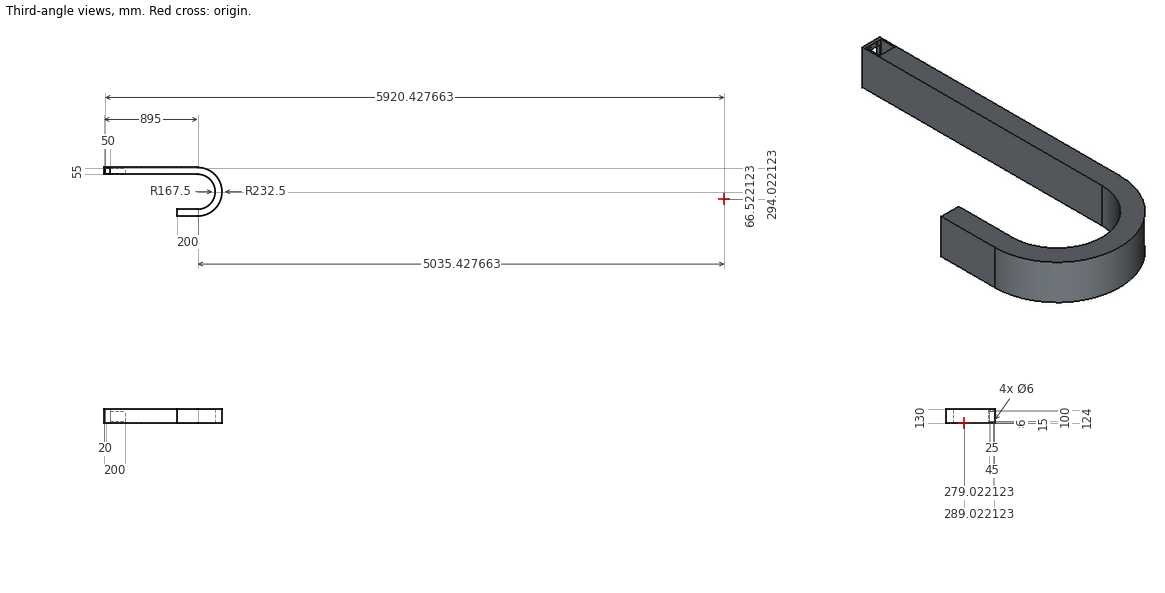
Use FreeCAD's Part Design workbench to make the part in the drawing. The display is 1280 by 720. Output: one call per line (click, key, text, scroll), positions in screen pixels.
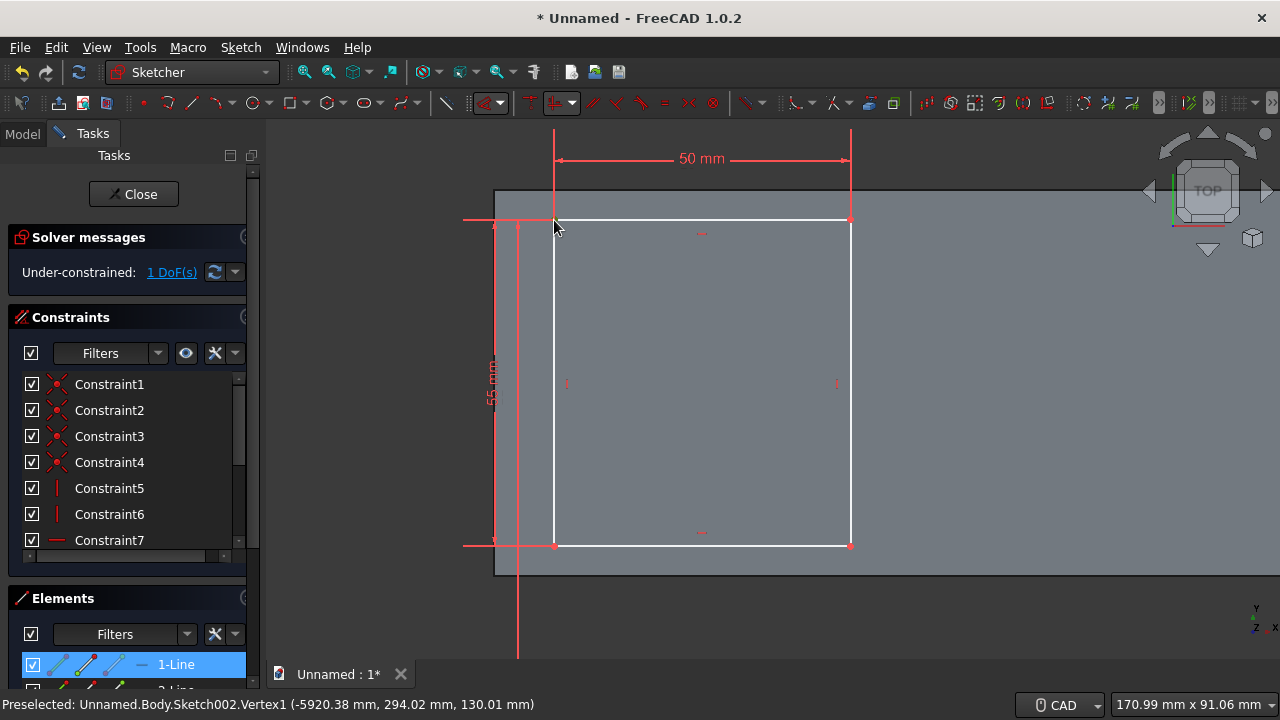
key(l)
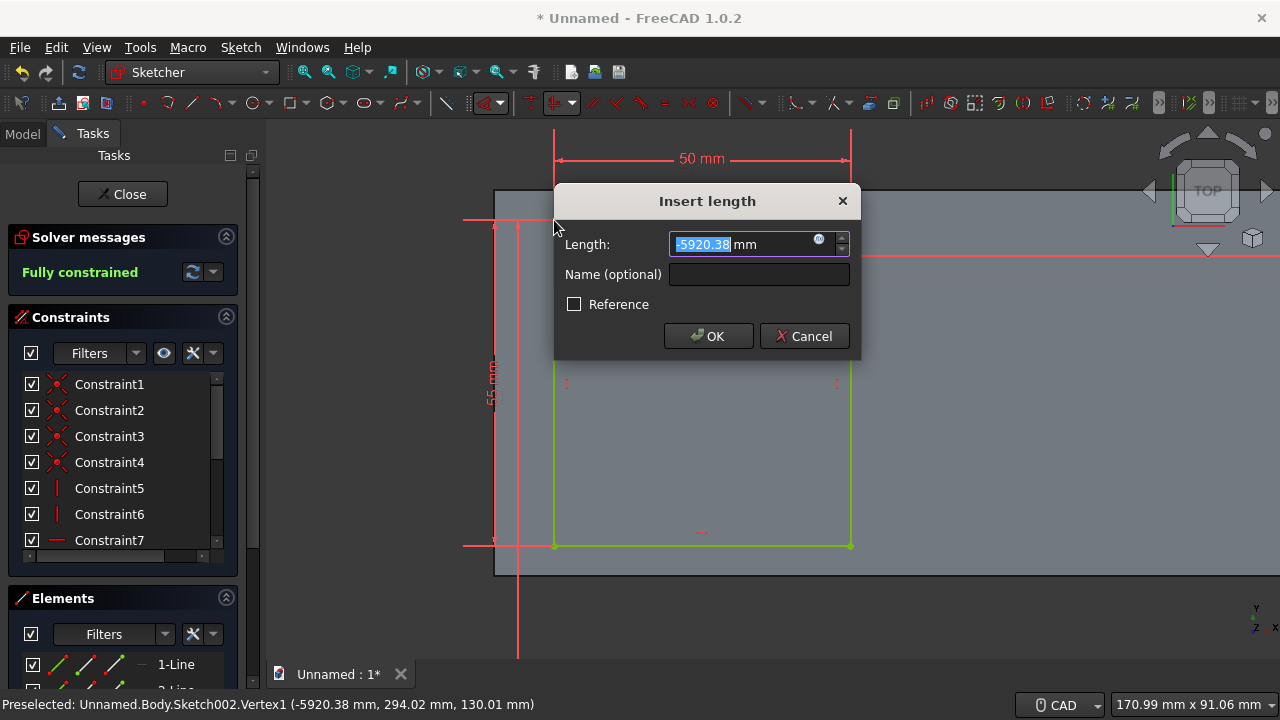
text(-5920.427663)
key(Return)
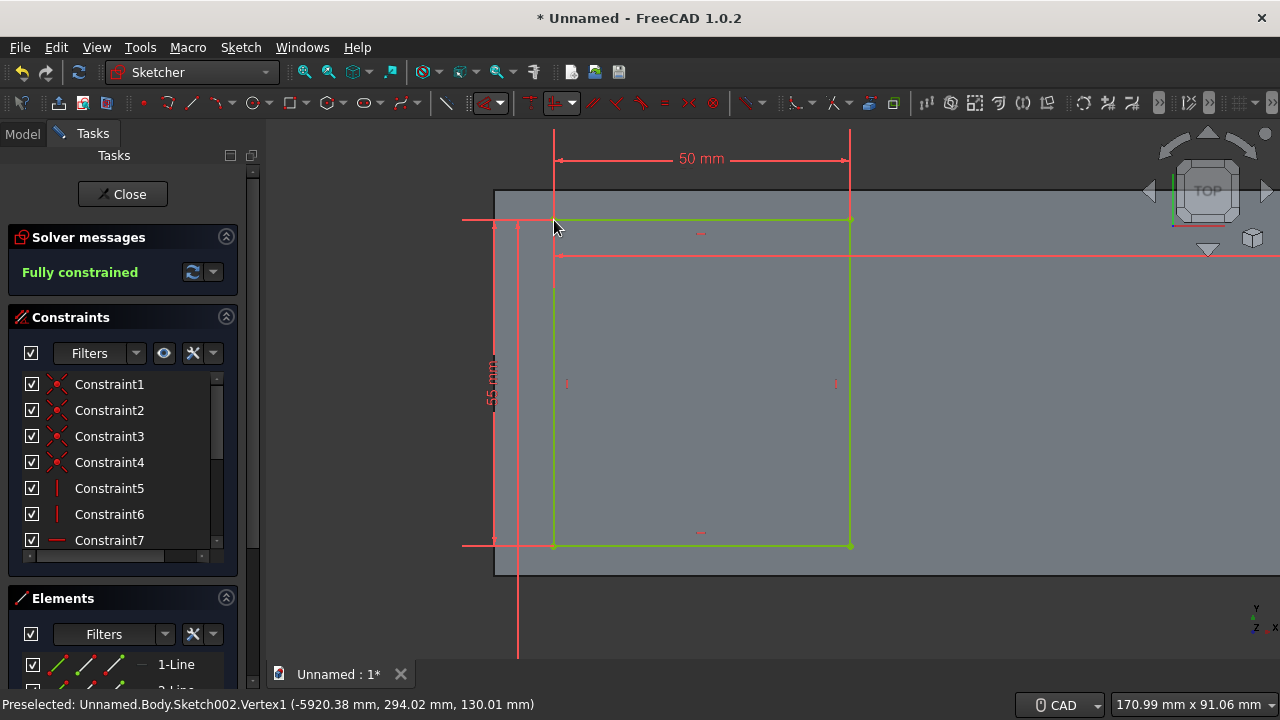
click(123, 194)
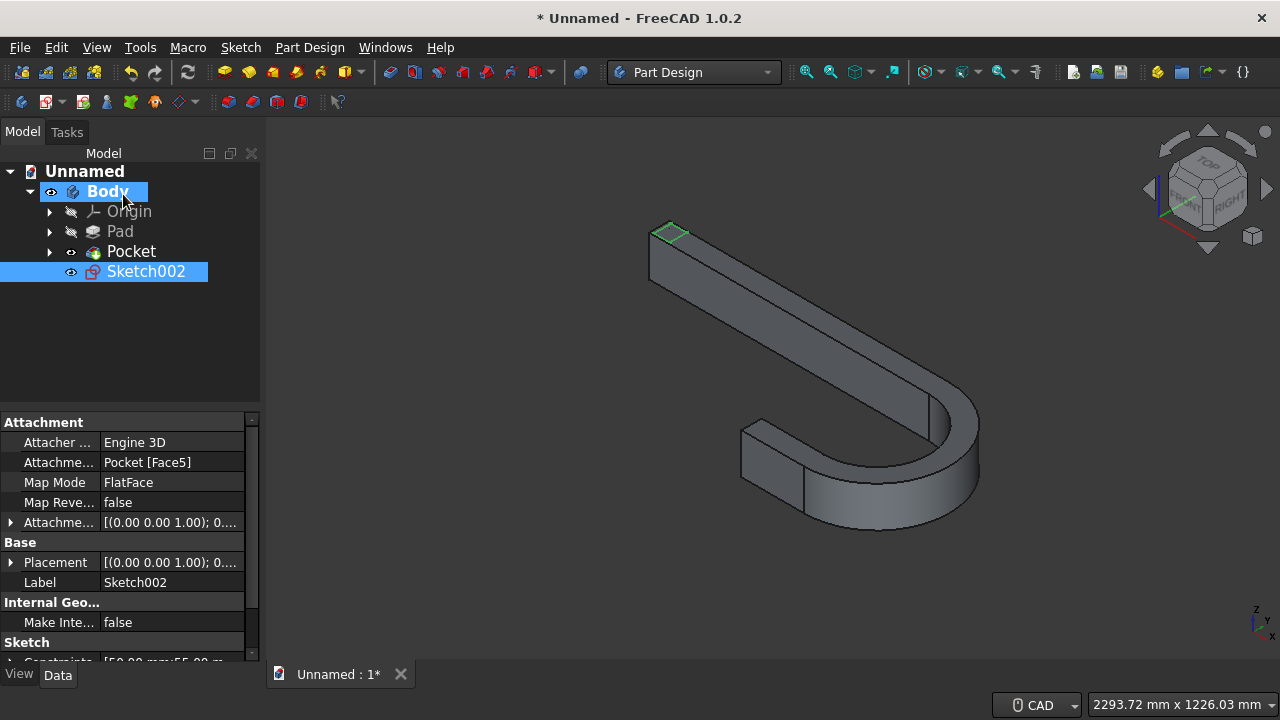
click(392, 72)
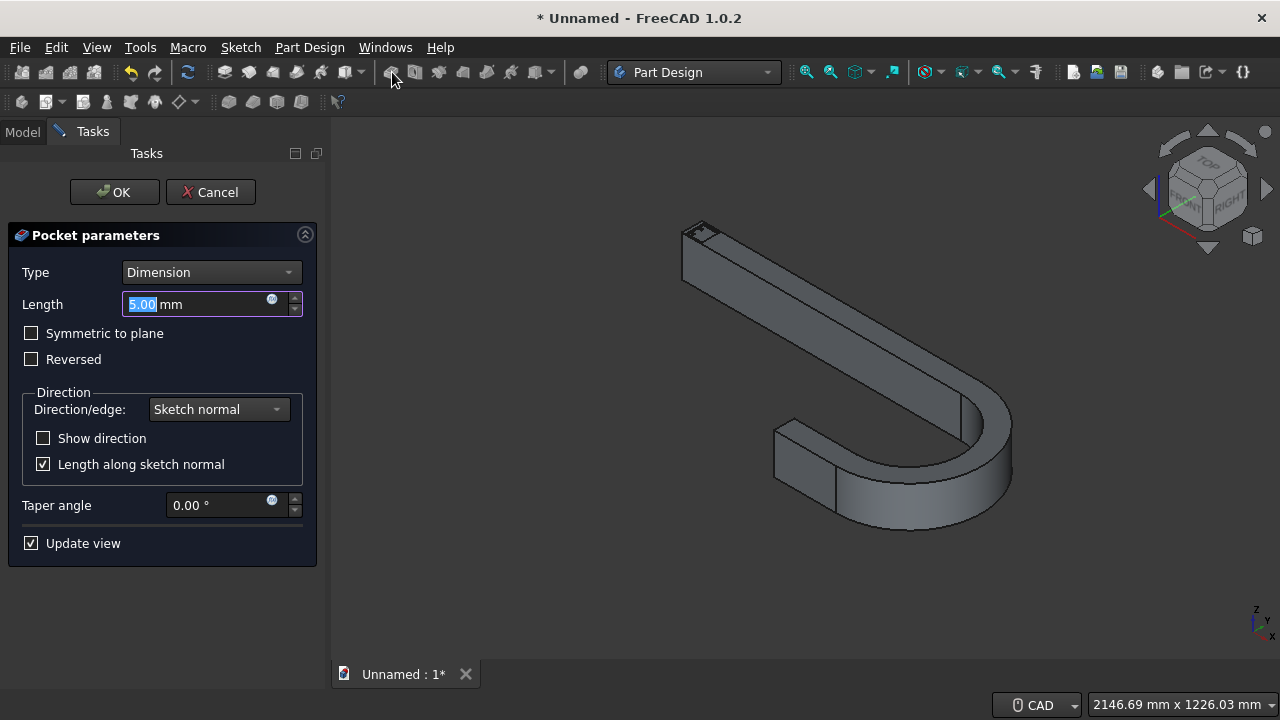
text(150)
key(Tab)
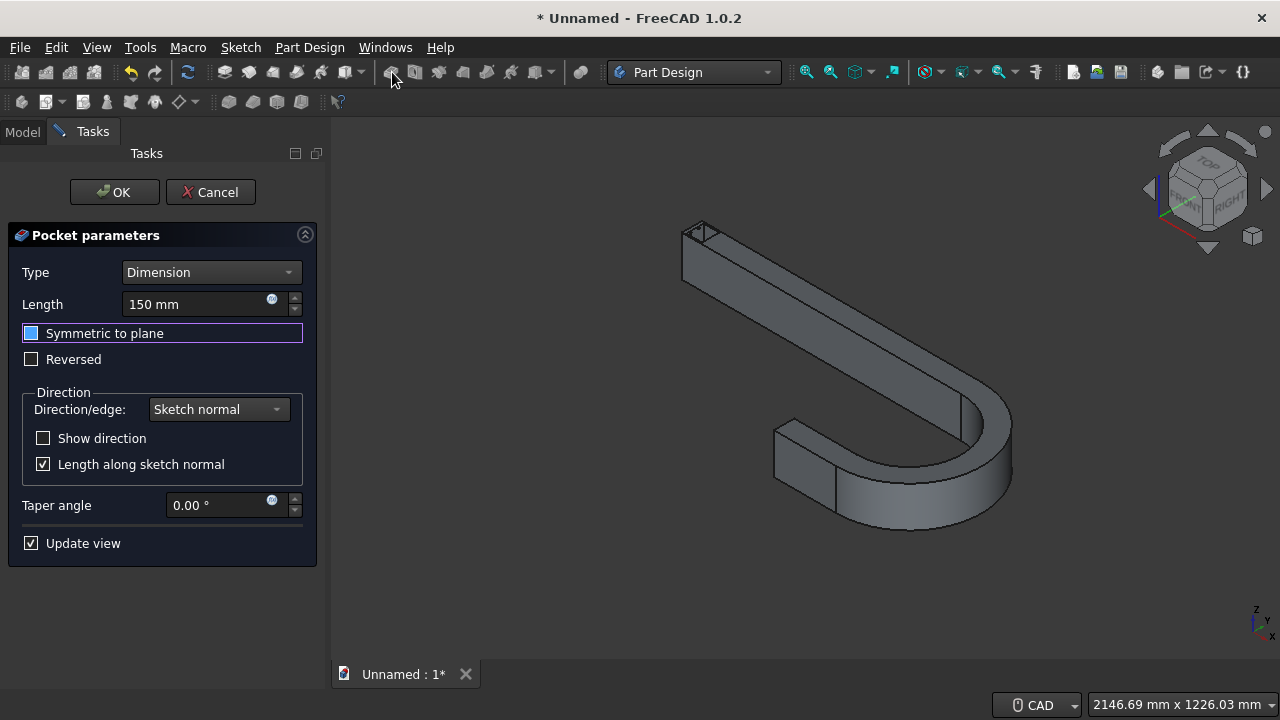
click(115, 192)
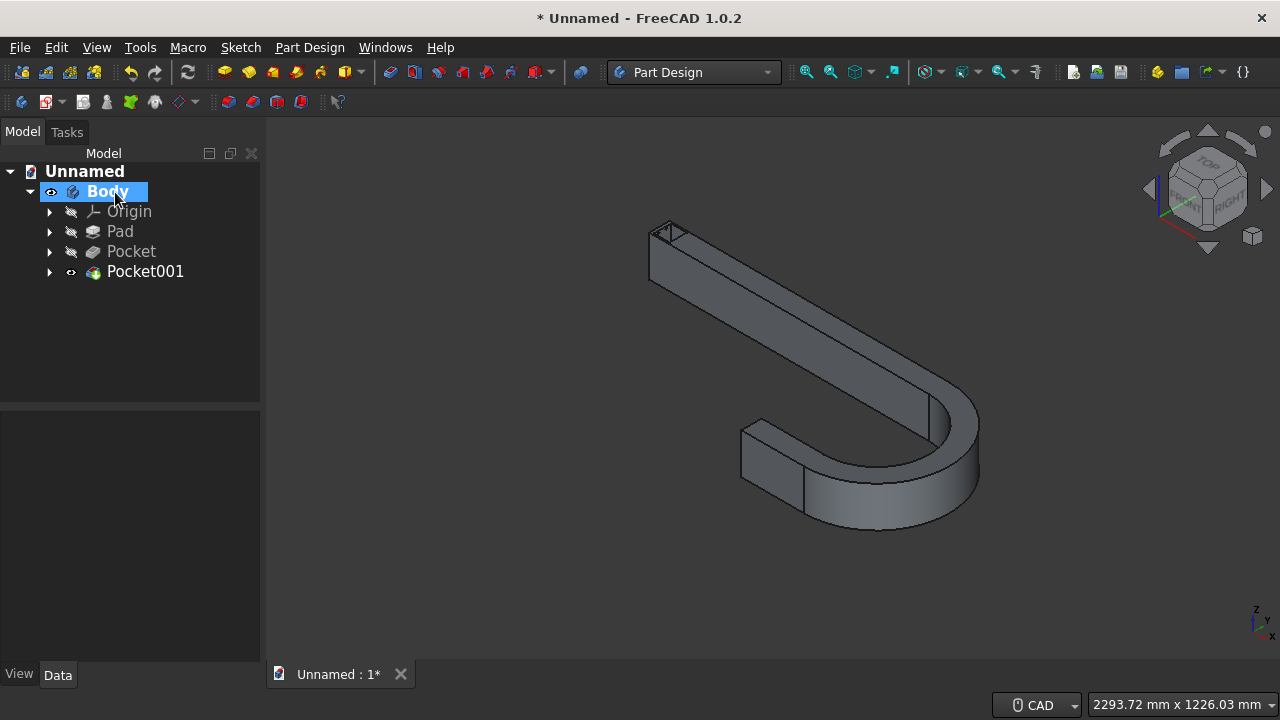
key(6)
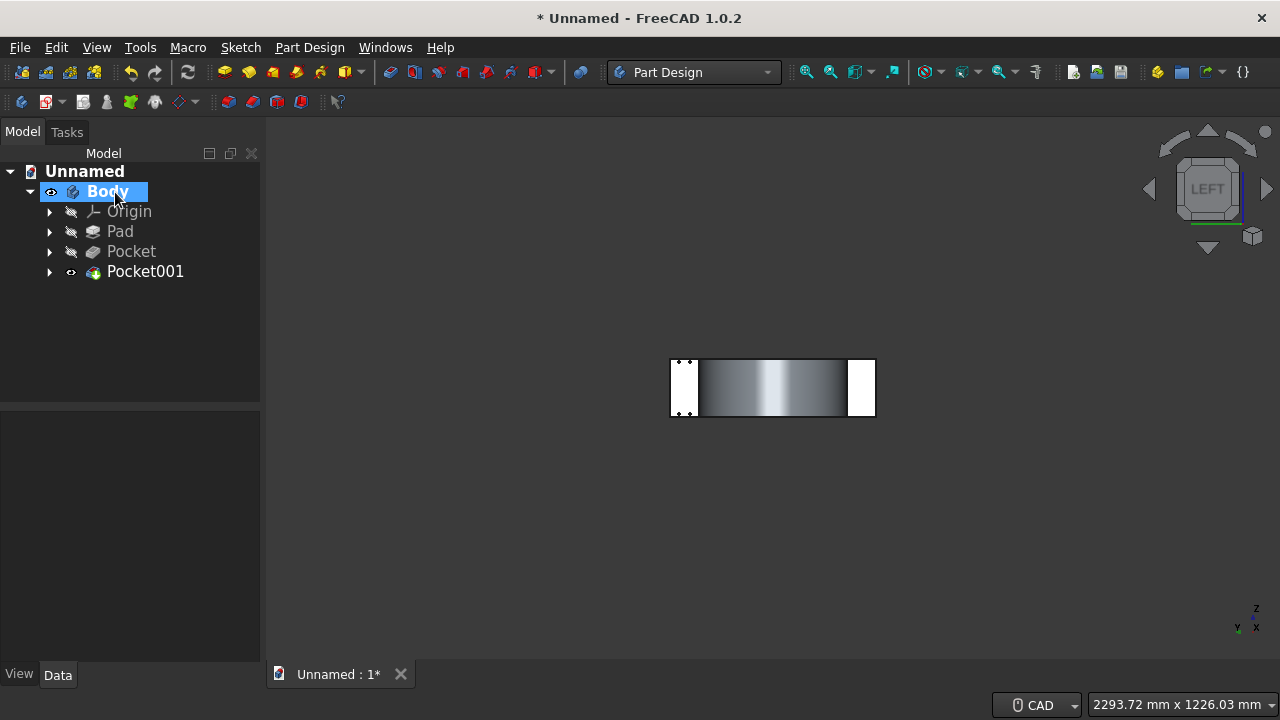
key(v)
key(f)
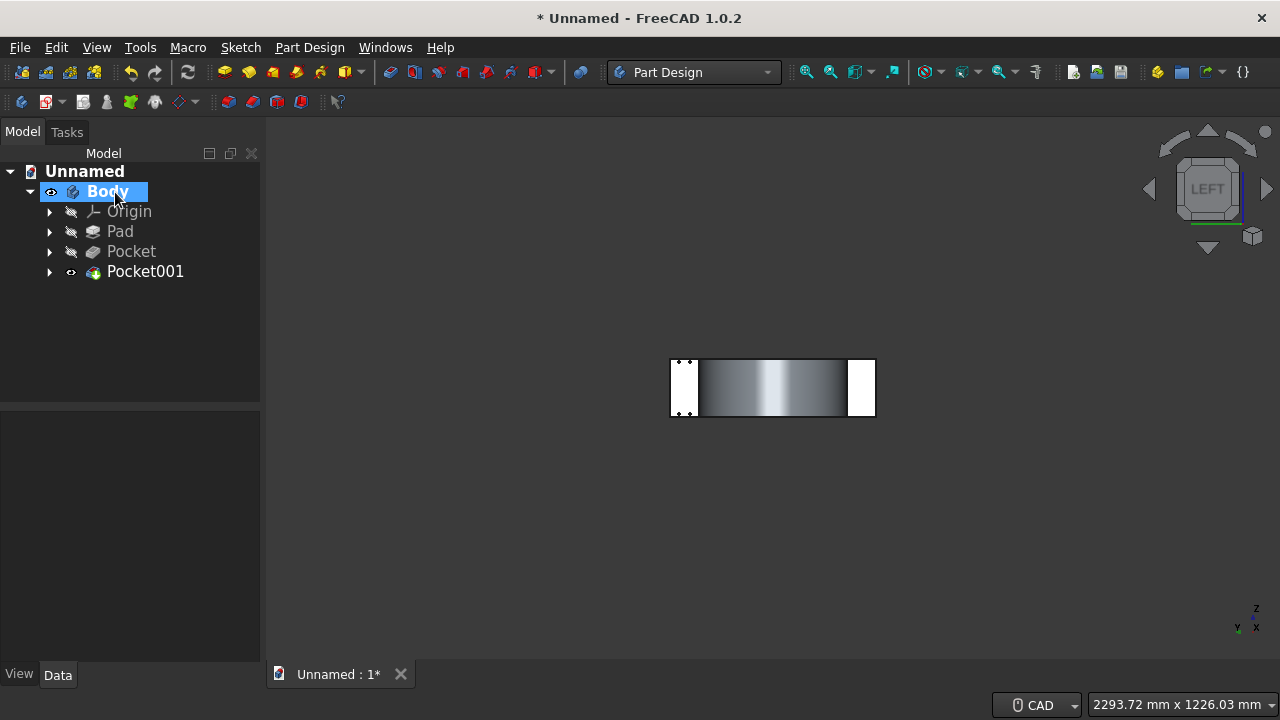
click(685, 379)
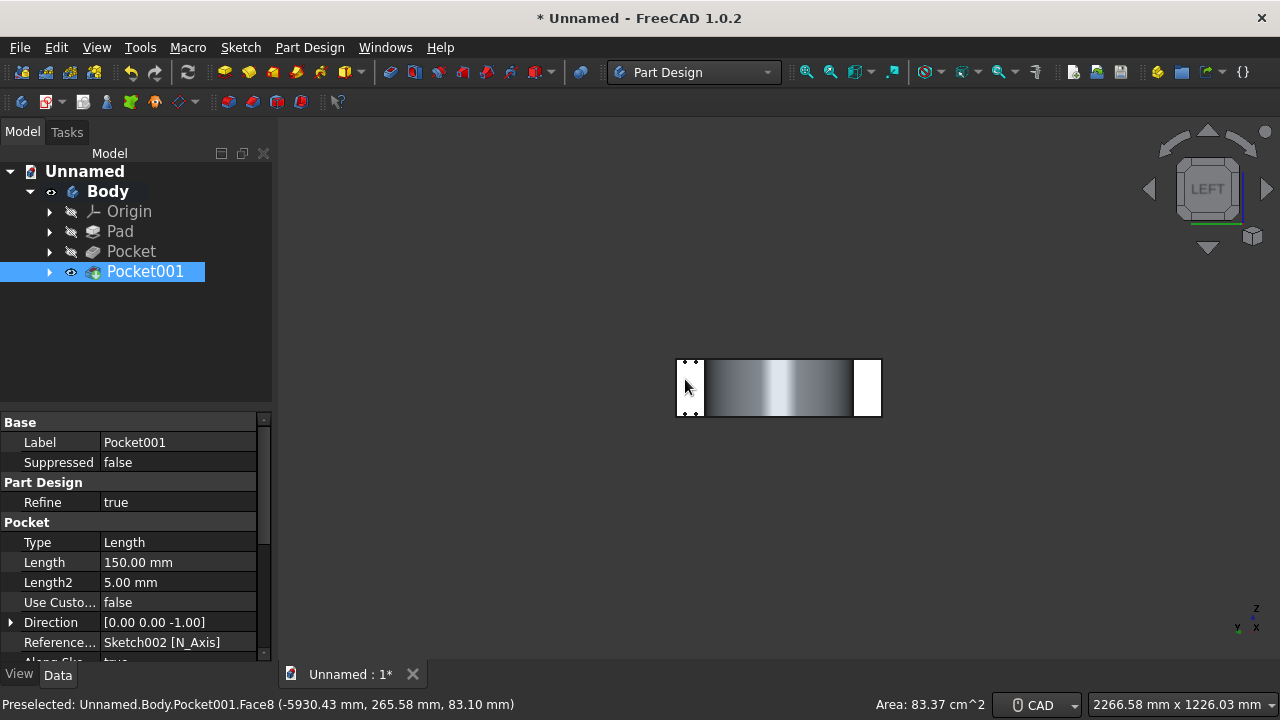
click(46, 102)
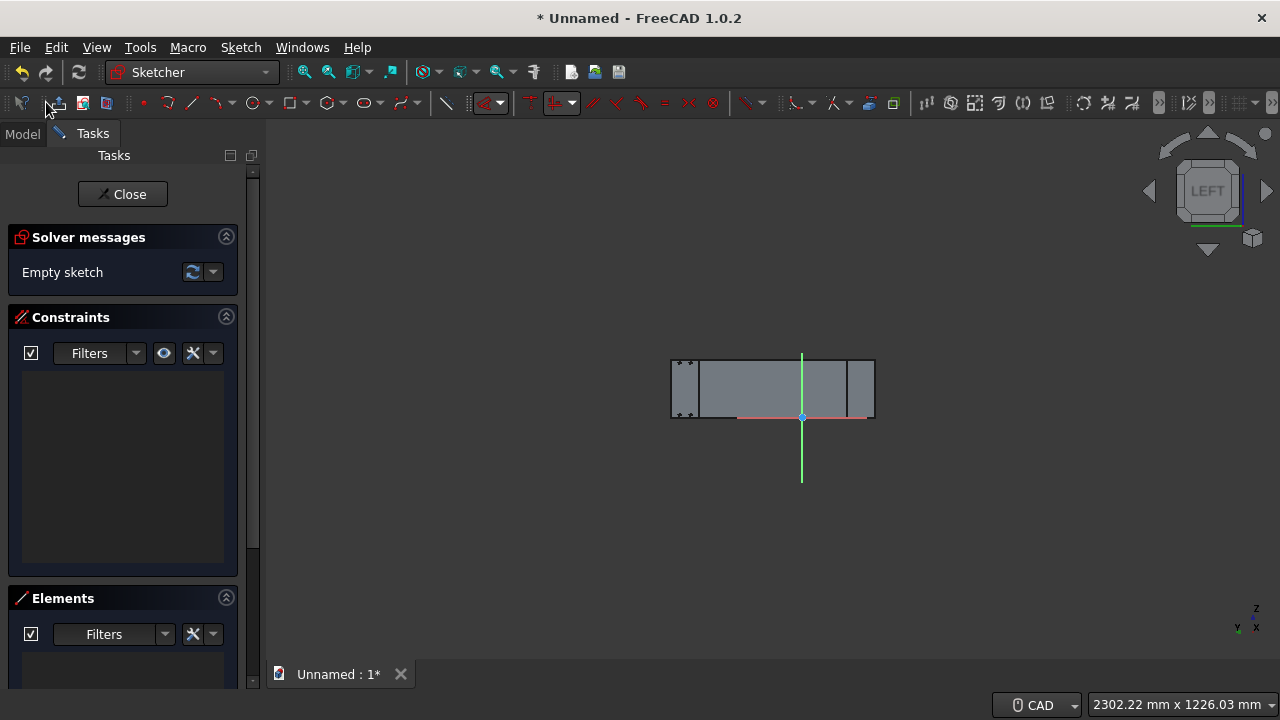
scroll(682, 389, up, 10)